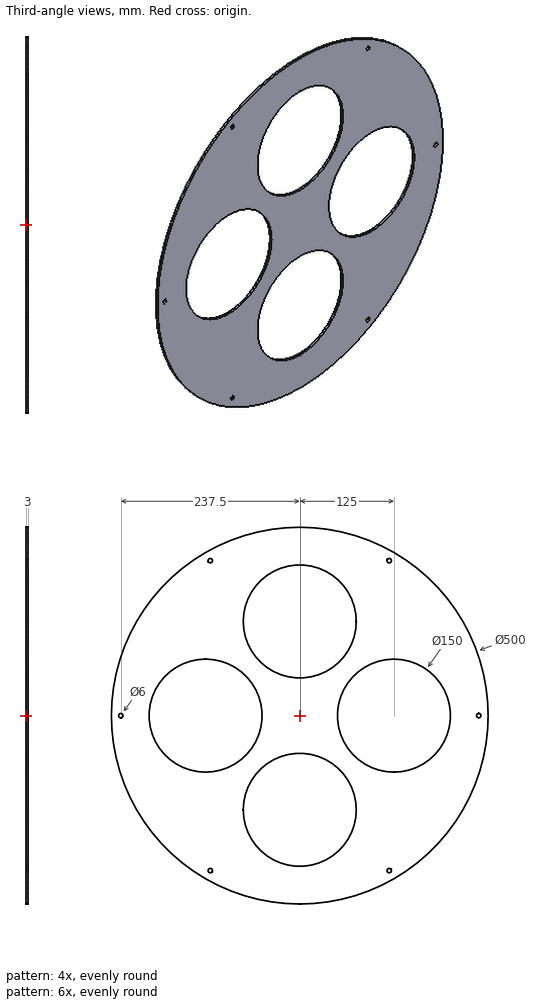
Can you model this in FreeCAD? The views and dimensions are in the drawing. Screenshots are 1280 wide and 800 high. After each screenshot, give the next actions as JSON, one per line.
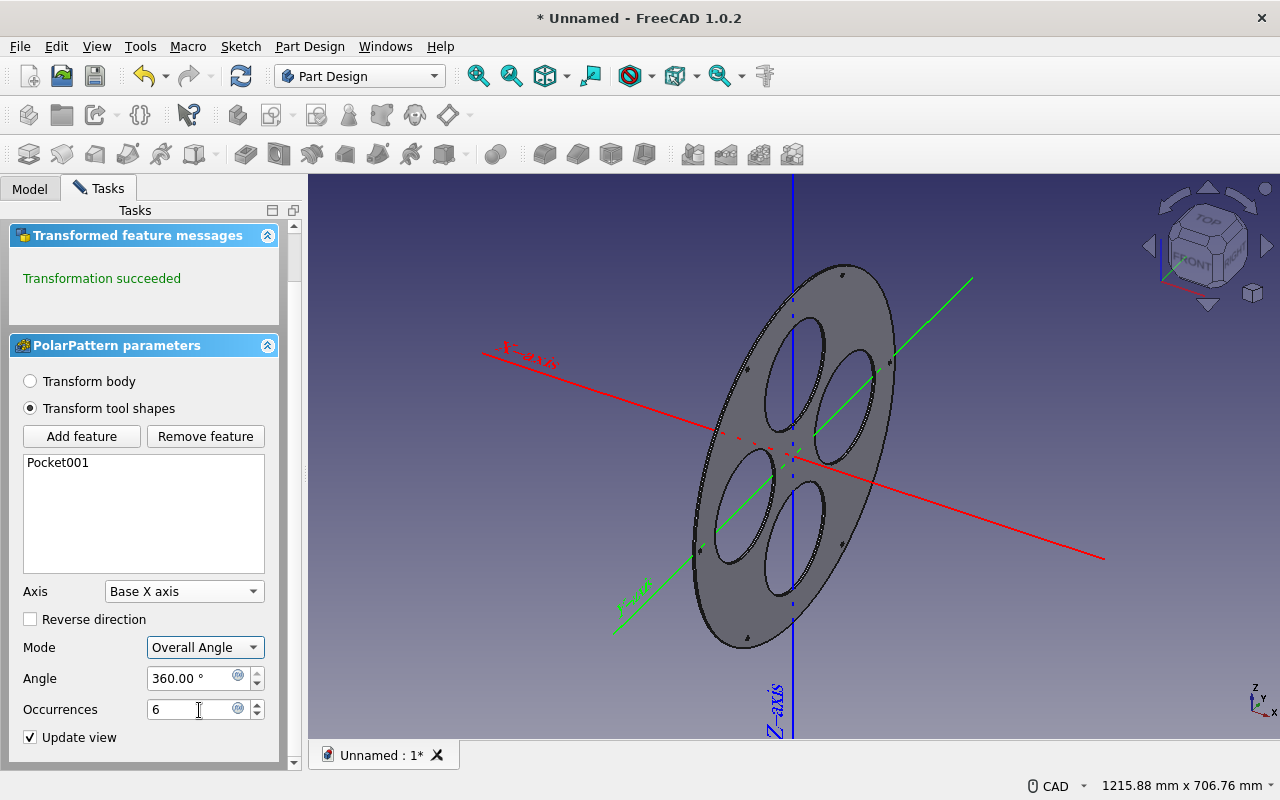
{"action": "scroll", "coordinate": [294, 495], "scroll_direction": "up", "scroll_amount": 2}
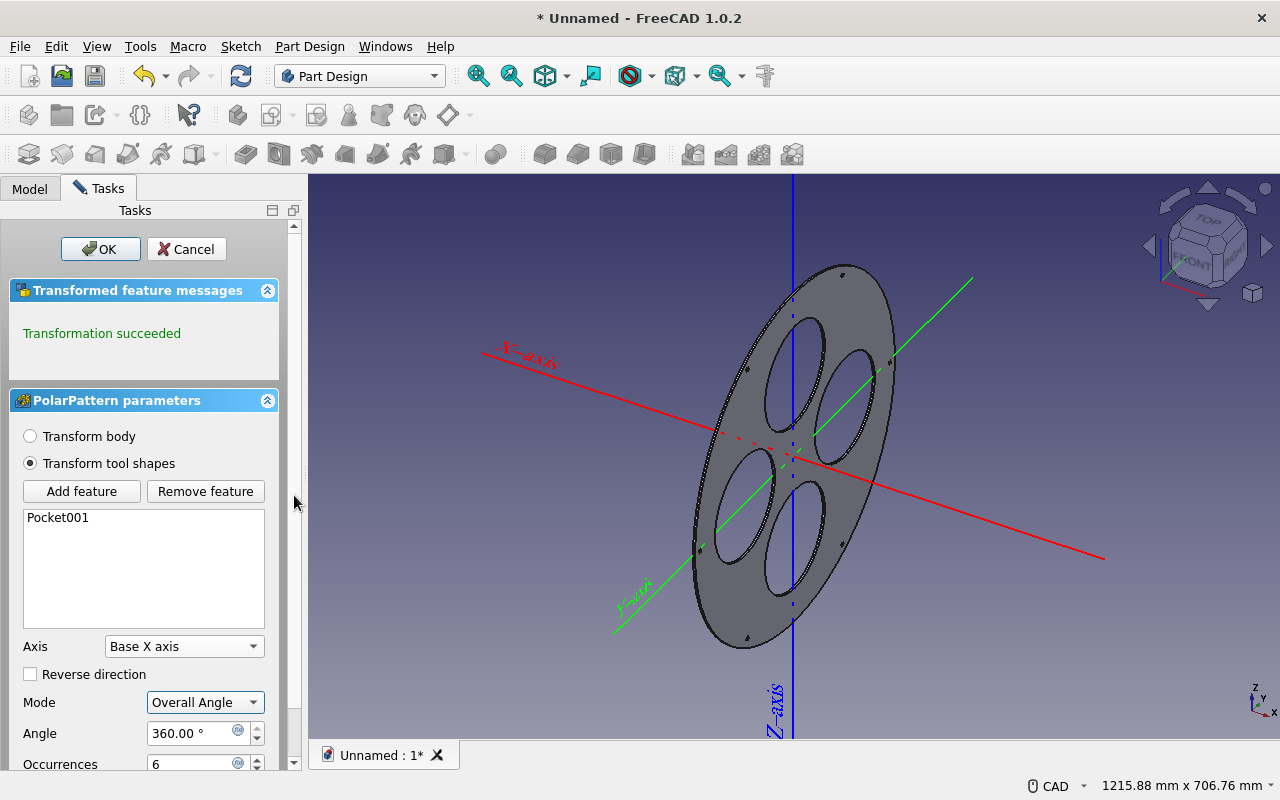
{"action": "left_click", "coordinate": [101, 249]}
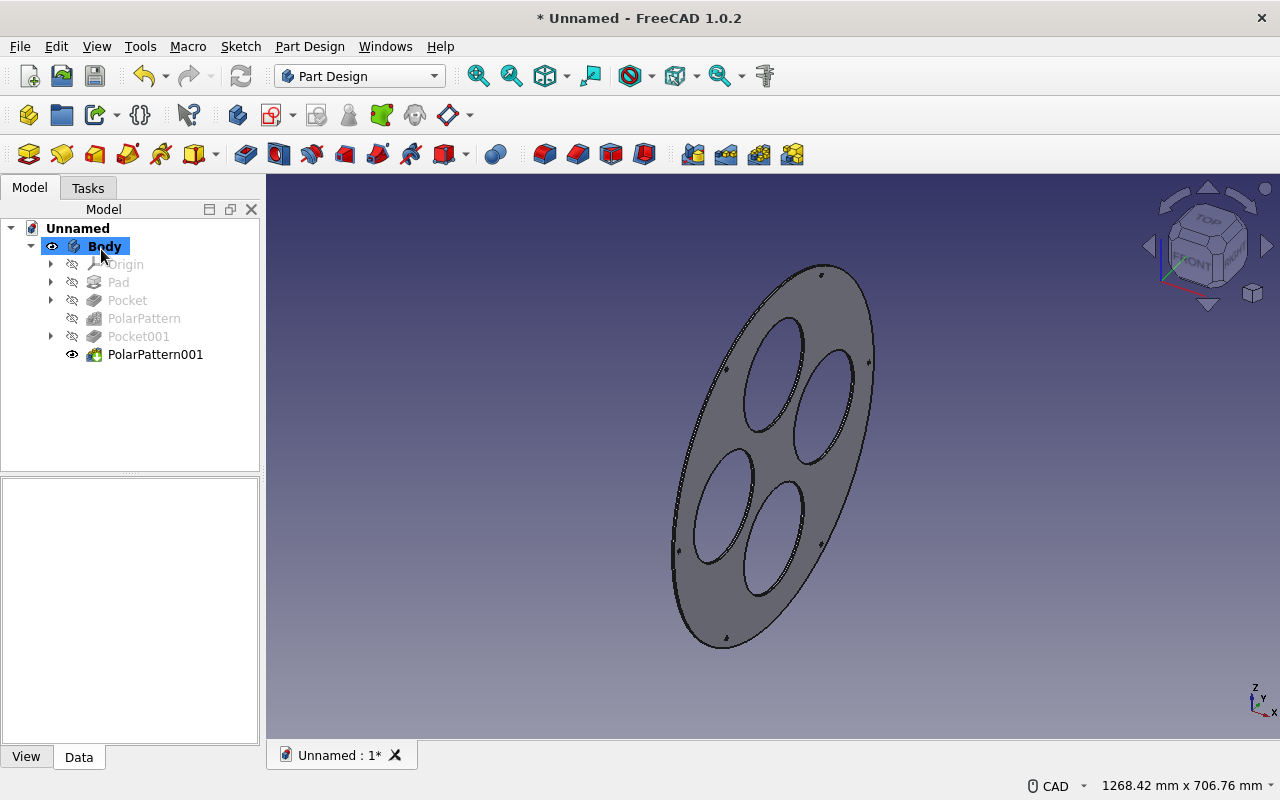
{"action": "key", "text": "0"}